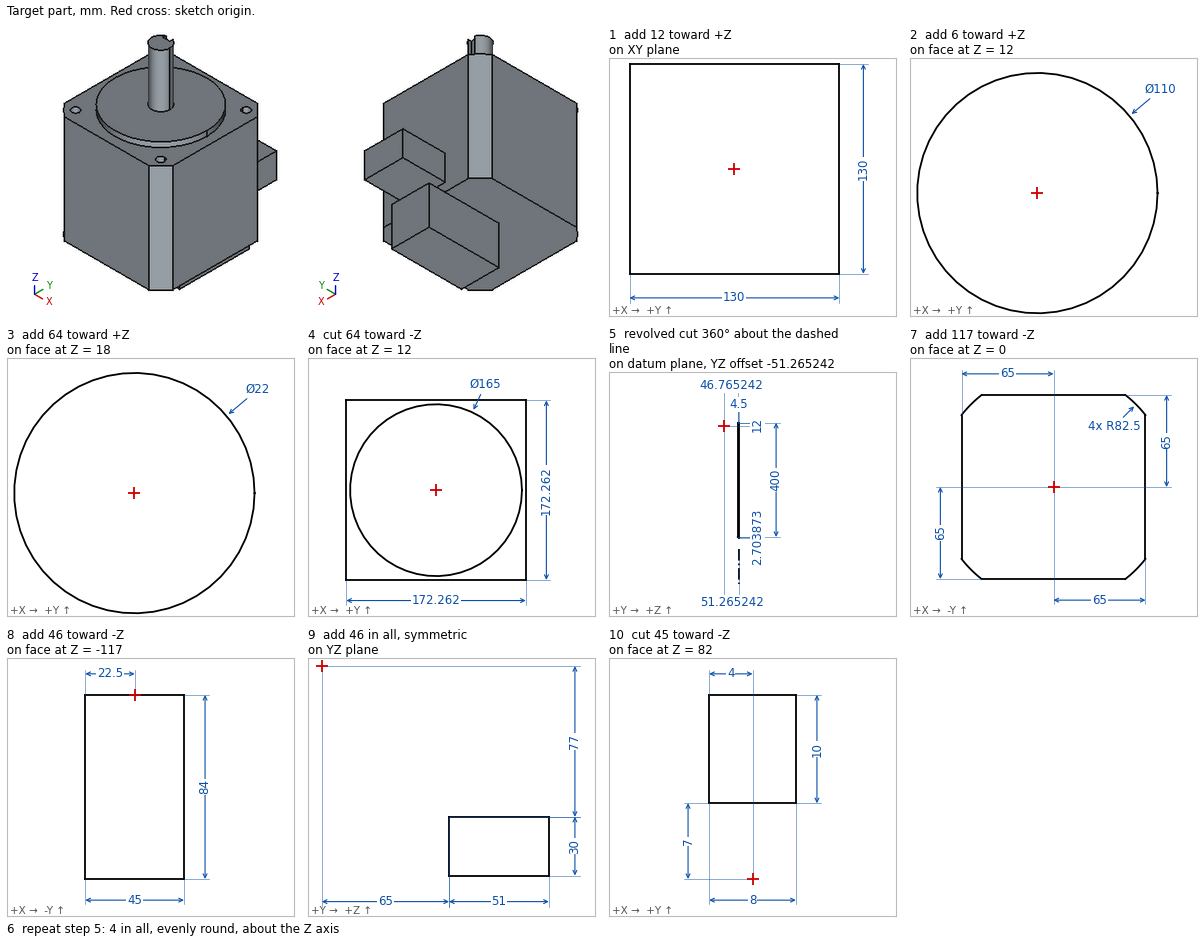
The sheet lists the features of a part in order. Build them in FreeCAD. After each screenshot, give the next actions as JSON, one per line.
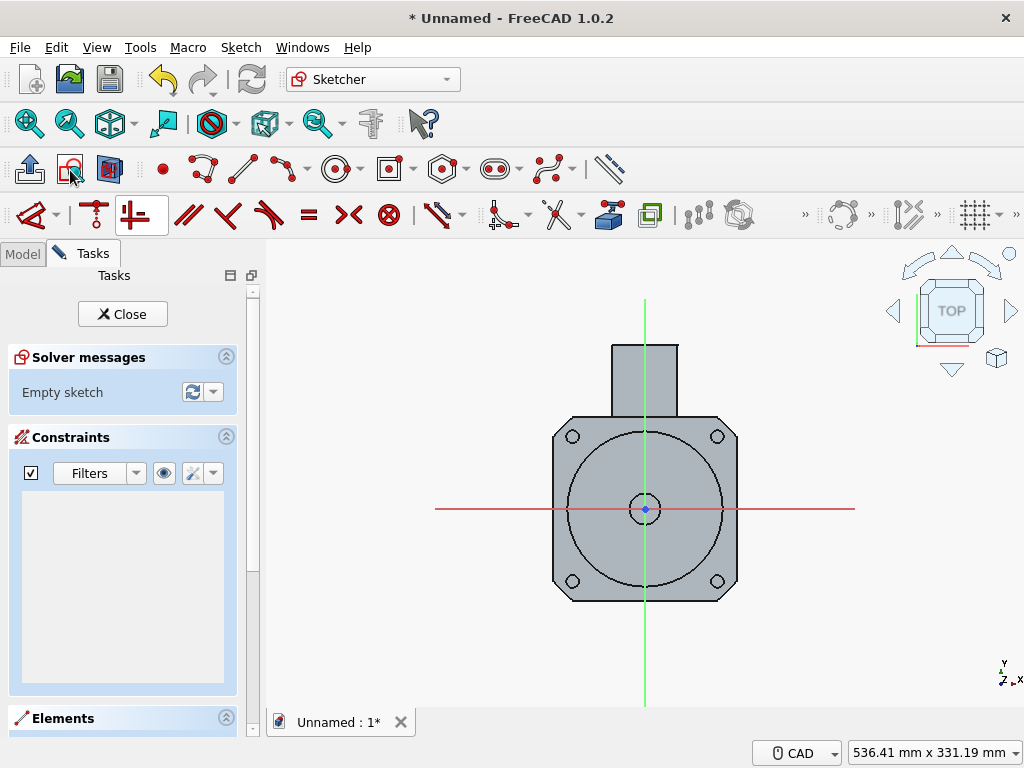
{"action": "scroll", "coordinate": [652, 499], "scroll_direction": "up", "scroll_amount": 12}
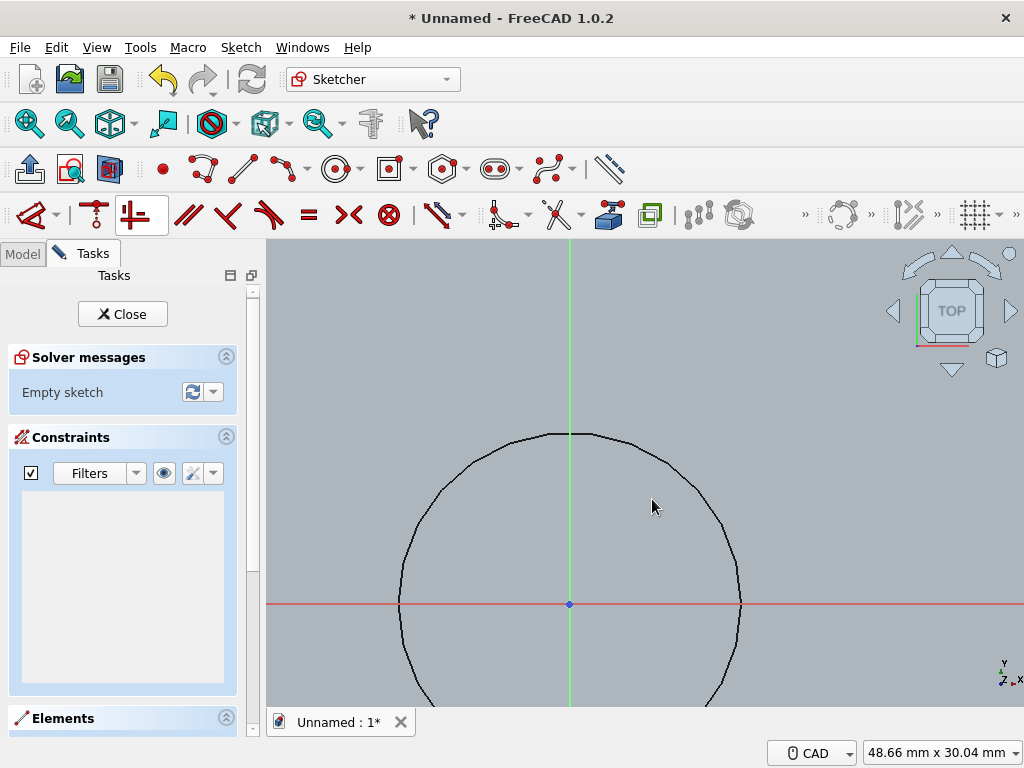
{"action": "left_click", "coordinate": [416, 170]}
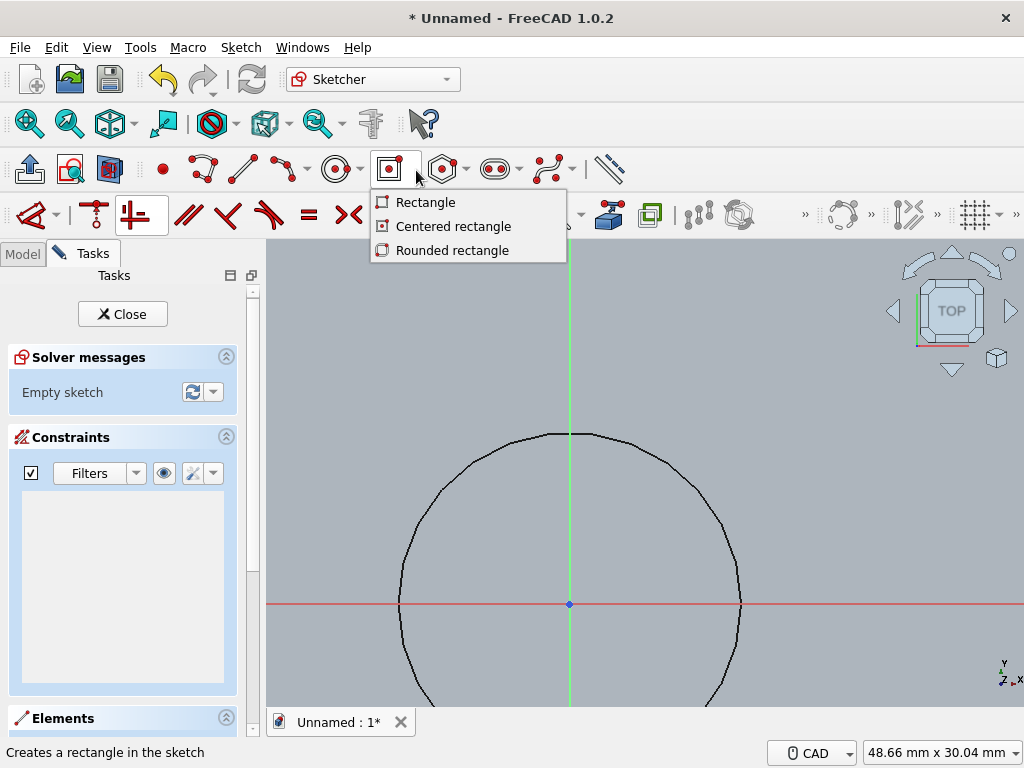
{"action": "left_click", "coordinate": [468, 202]}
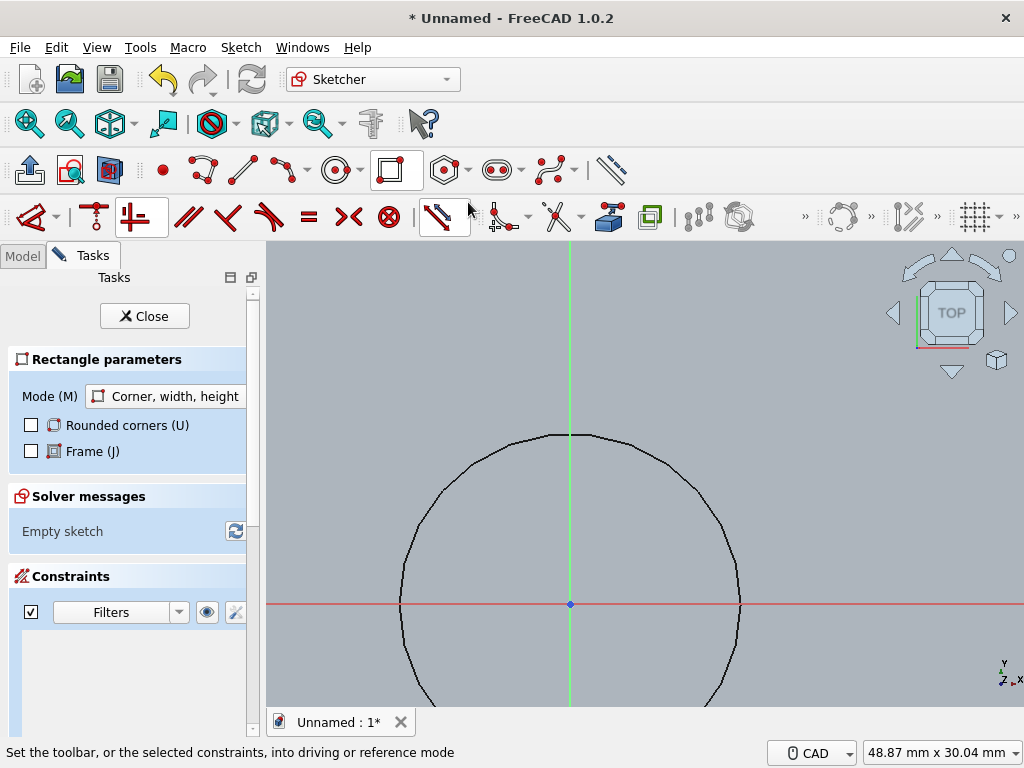
{"action": "left_click", "coordinate": [508, 341]}
{"action": "mouse_move", "coordinate": [632, 496]}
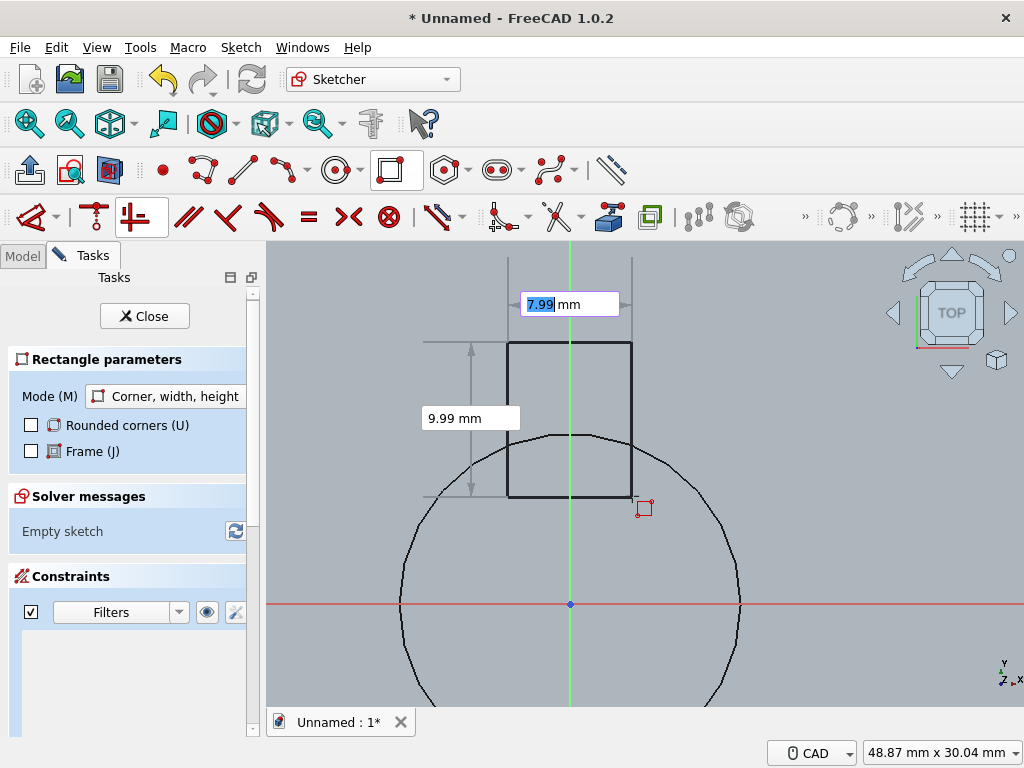
{"action": "type", "text": "8"}
{"action": "key", "text": "Tab"}
{"action": "type", "text": "10"}
{"action": "key", "text": "Return"}
{"action": "key", "text": "Escape"}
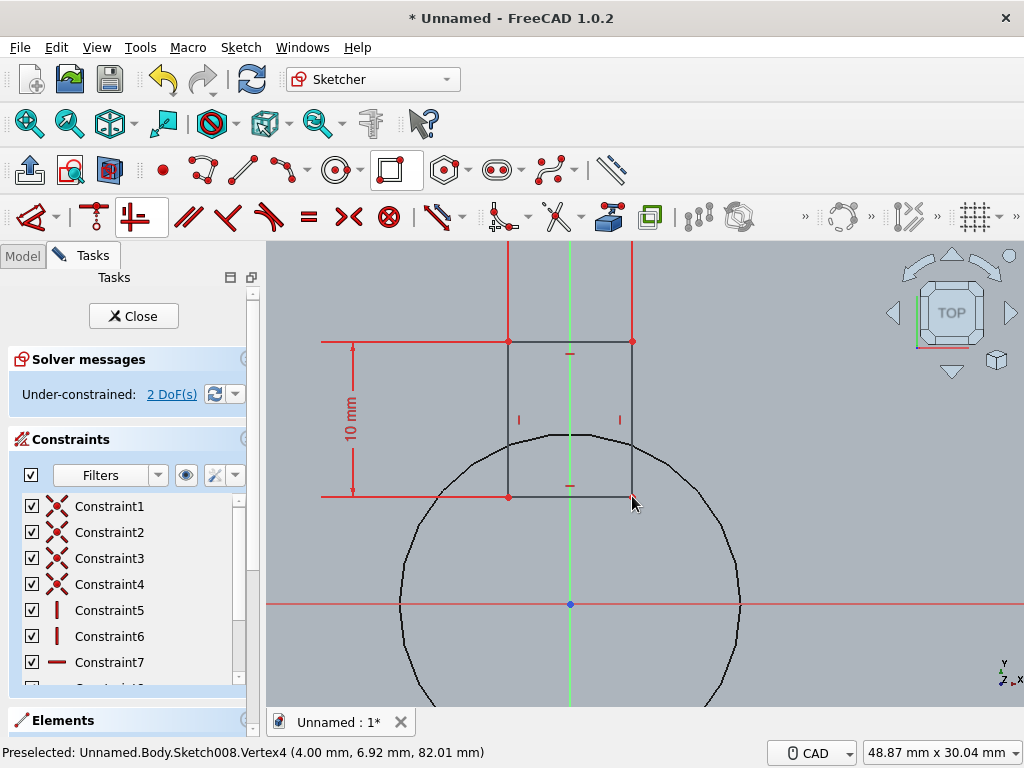
{"action": "left_click", "coordinate": [32, 218]}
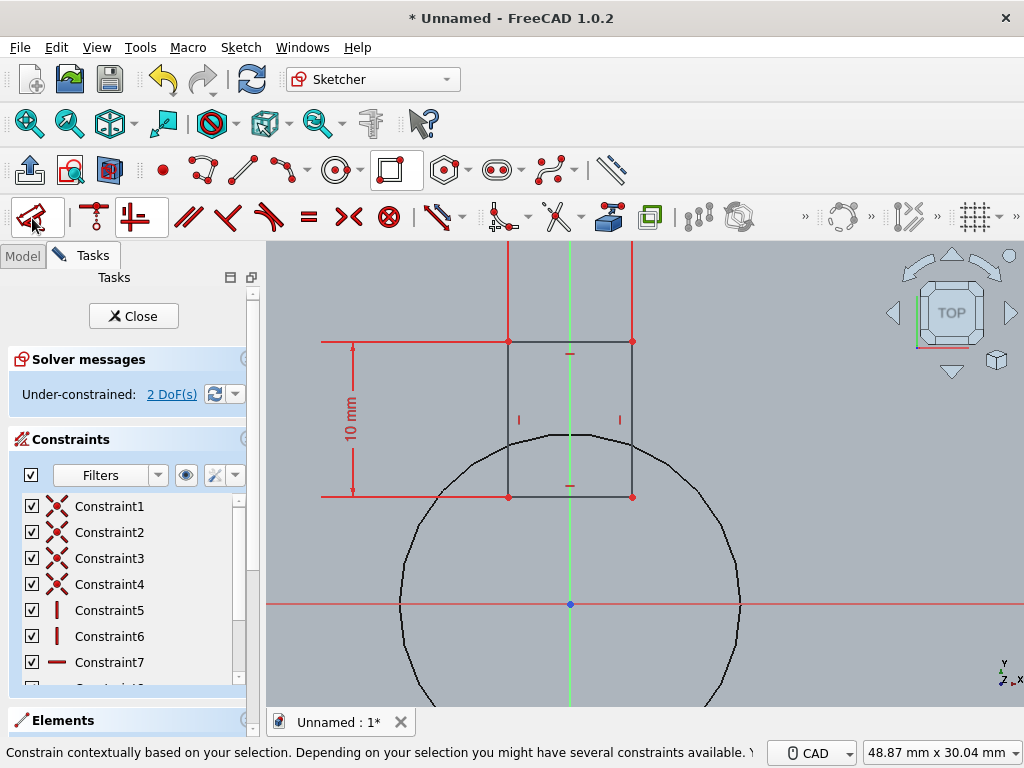
{"action": "left_click", "coordinate": [508, 342]}
{"action": "left_click", "coordinate": [539, 638]}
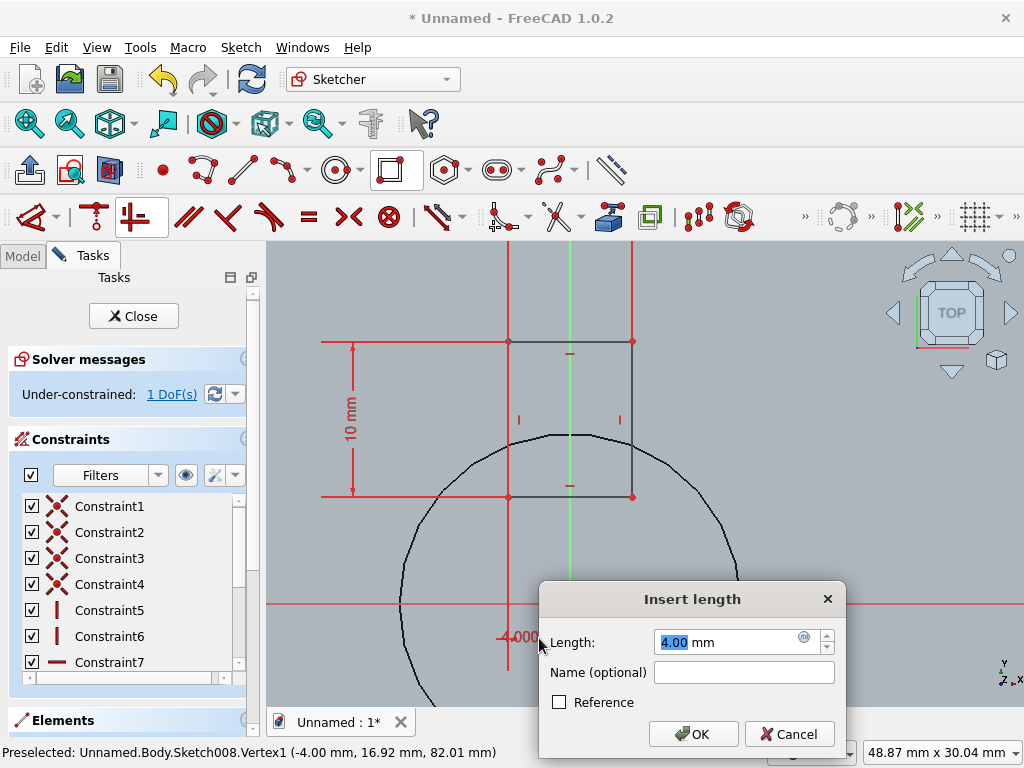
{"action": "type", "text": "4"}
{"action": "key", "text": "Return"}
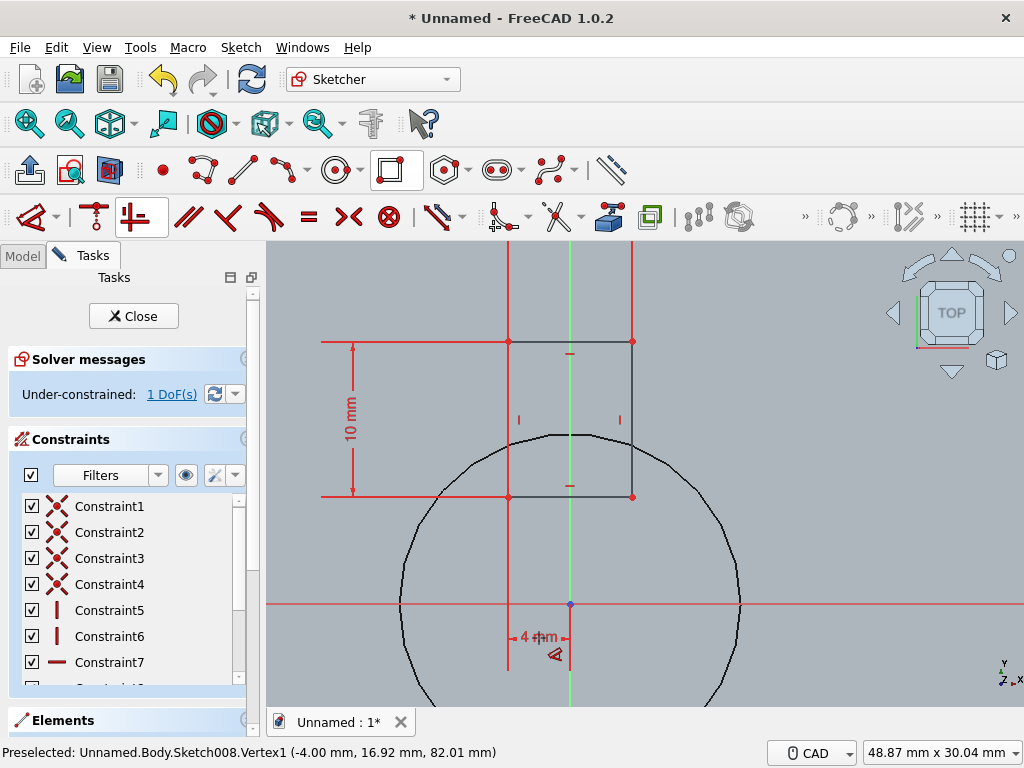
{"action": "left_click", "coordinate": [508, 497]}
{"action": "left_click", "coordinate": [474, 551]}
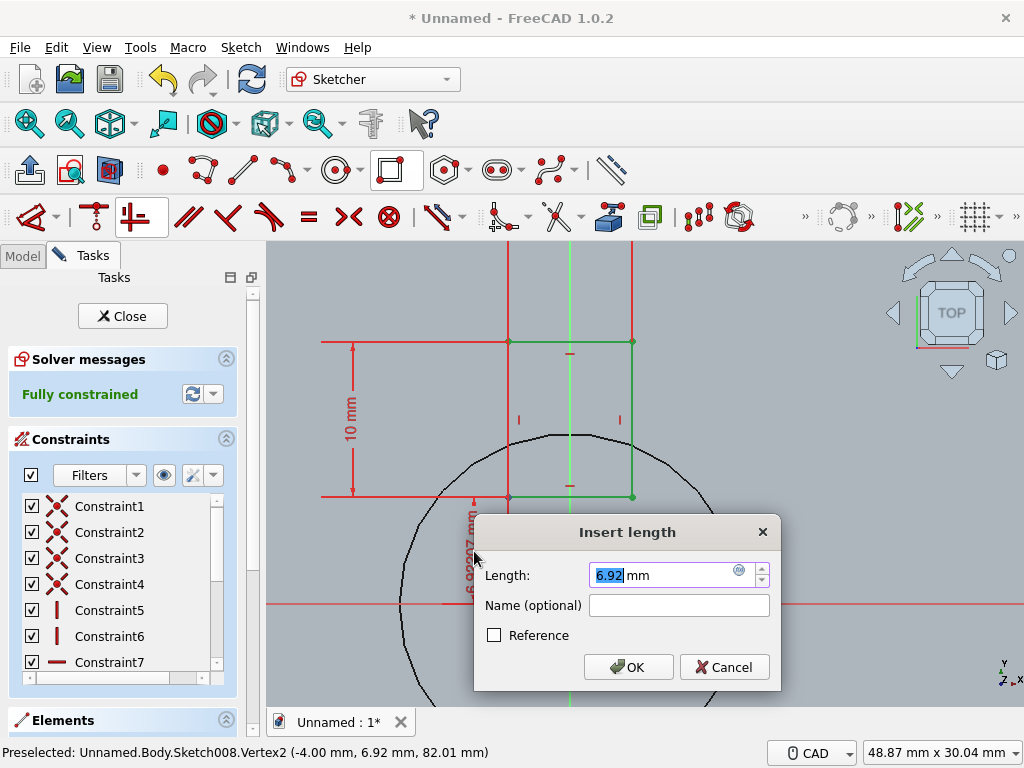
{"action": "type", "text": "7"}
{"action": "key", "text": "Return"}
{"action": "key", "text": "Escape"}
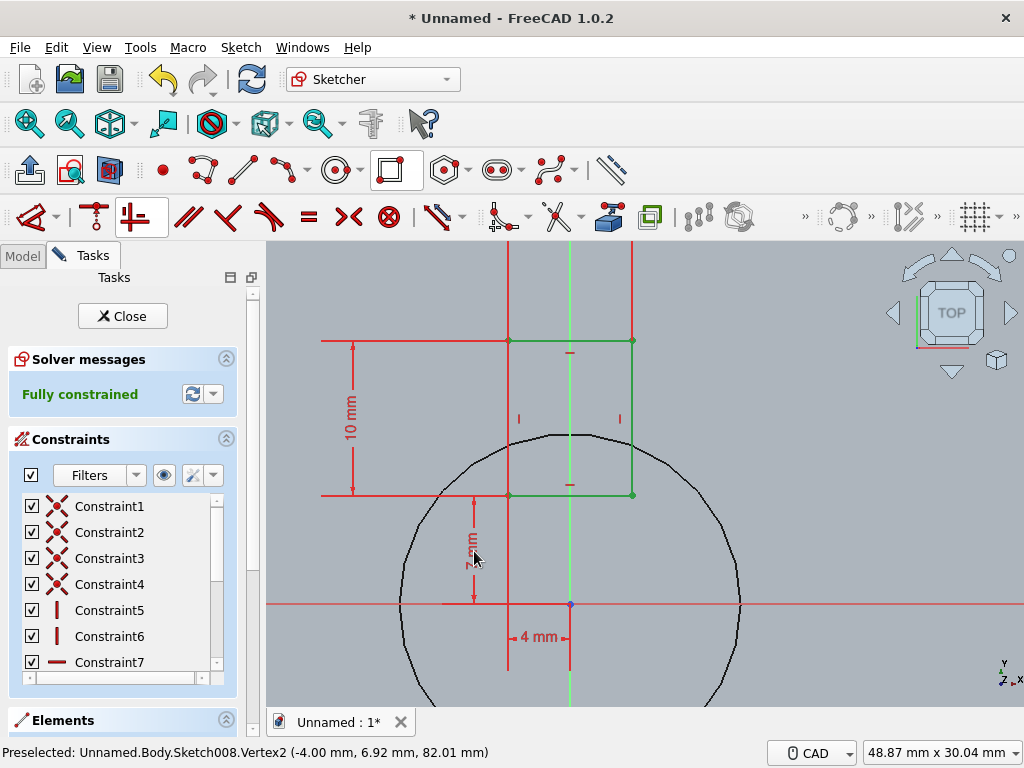
{"action": "left_click", "coordinate": [123, 316]}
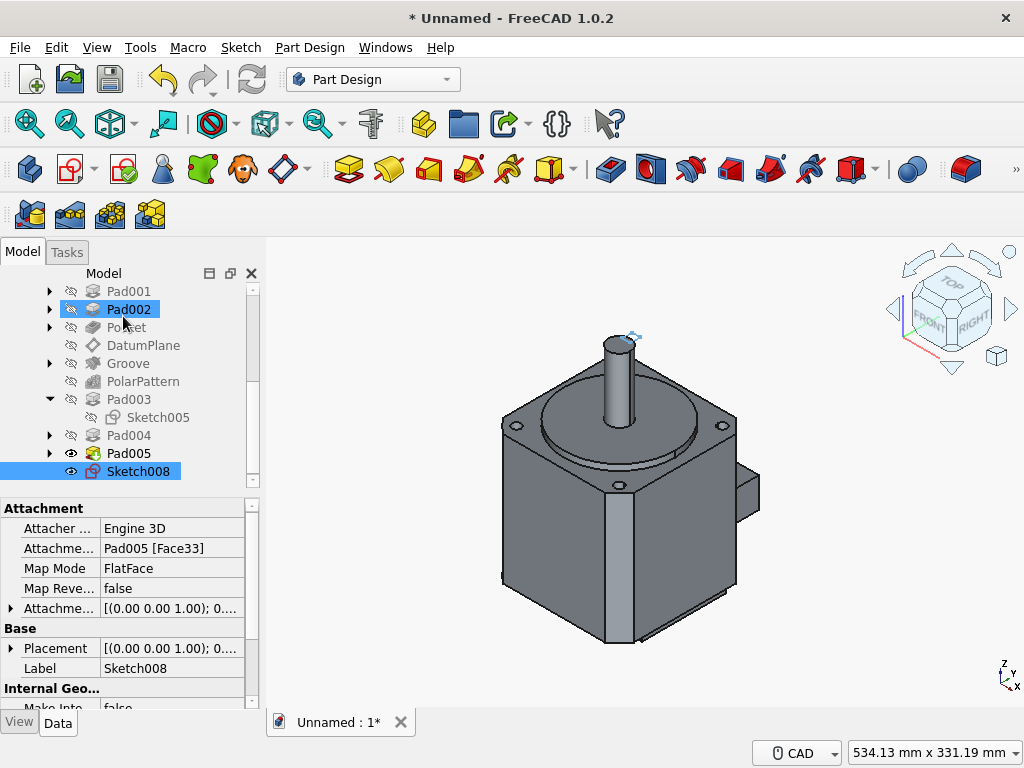
{"action": "left_click", "coordinate": [612, 170]}